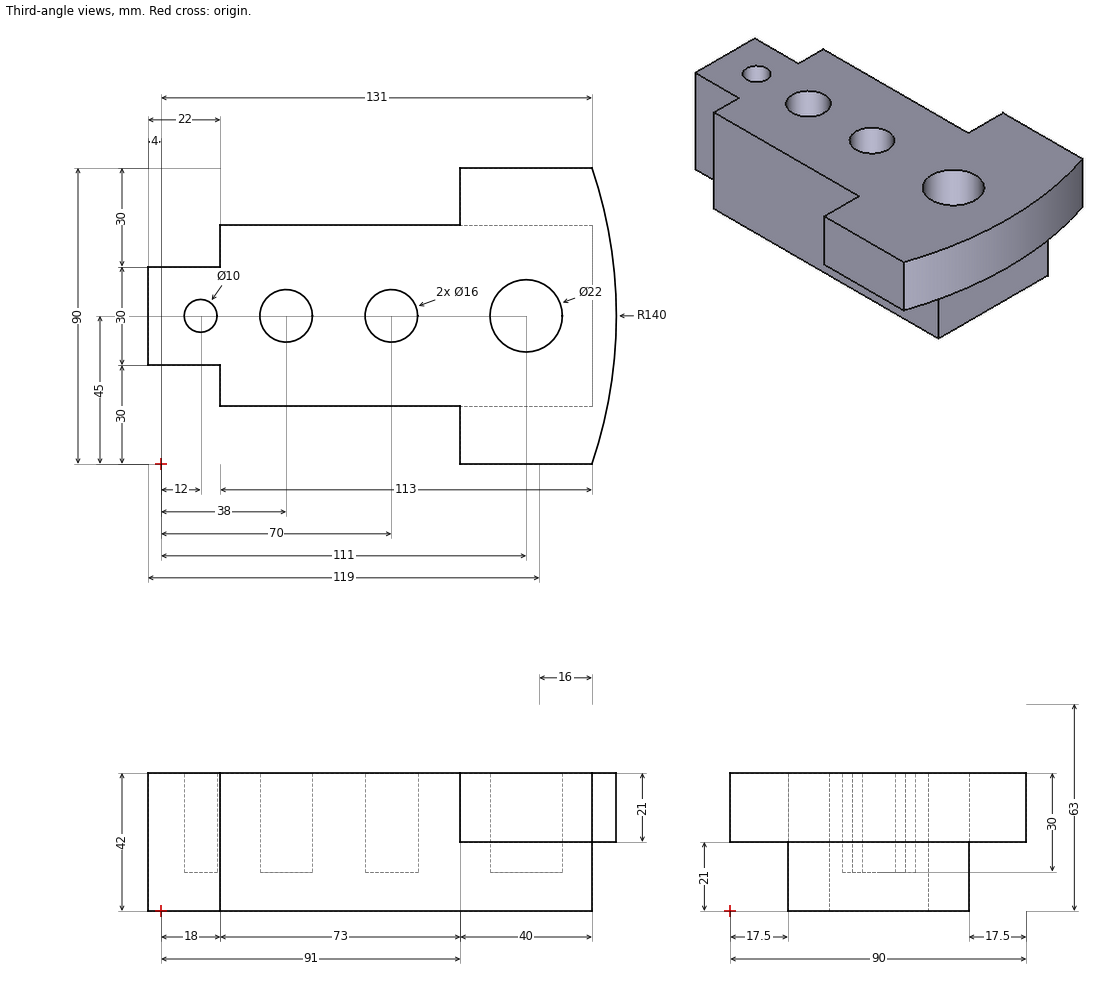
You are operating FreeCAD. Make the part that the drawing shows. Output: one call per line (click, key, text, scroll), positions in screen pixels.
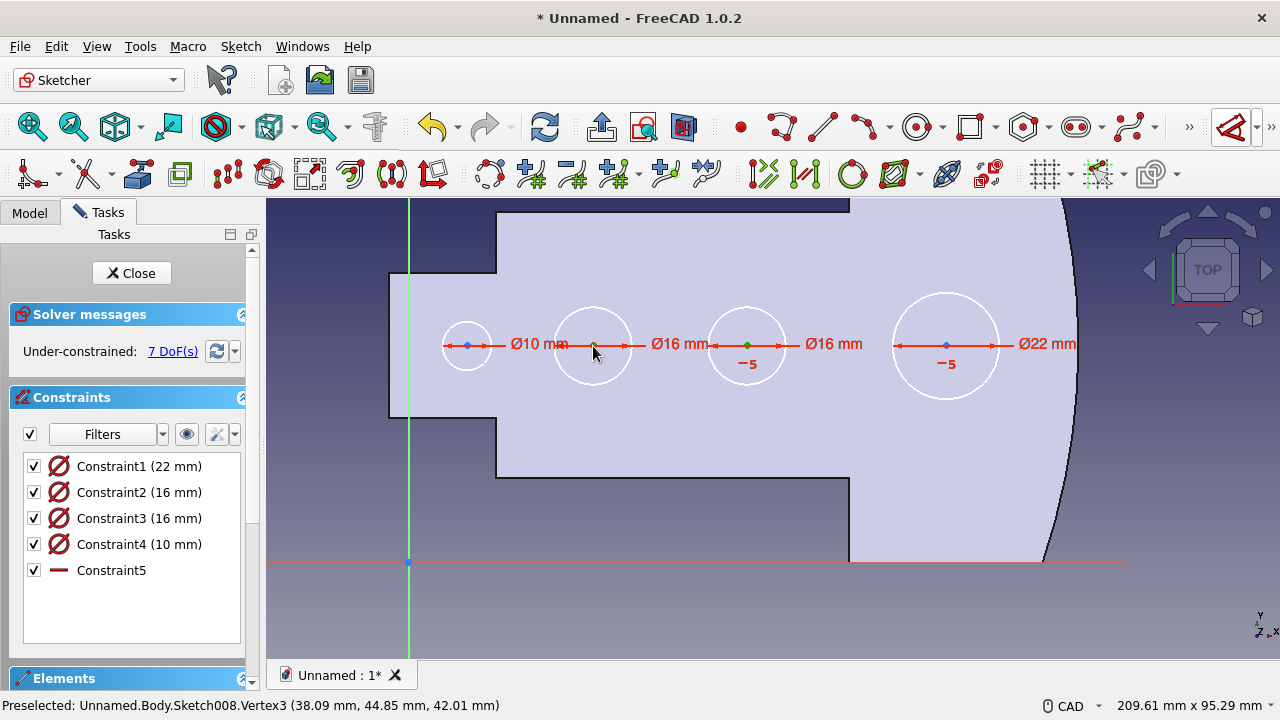
key(h)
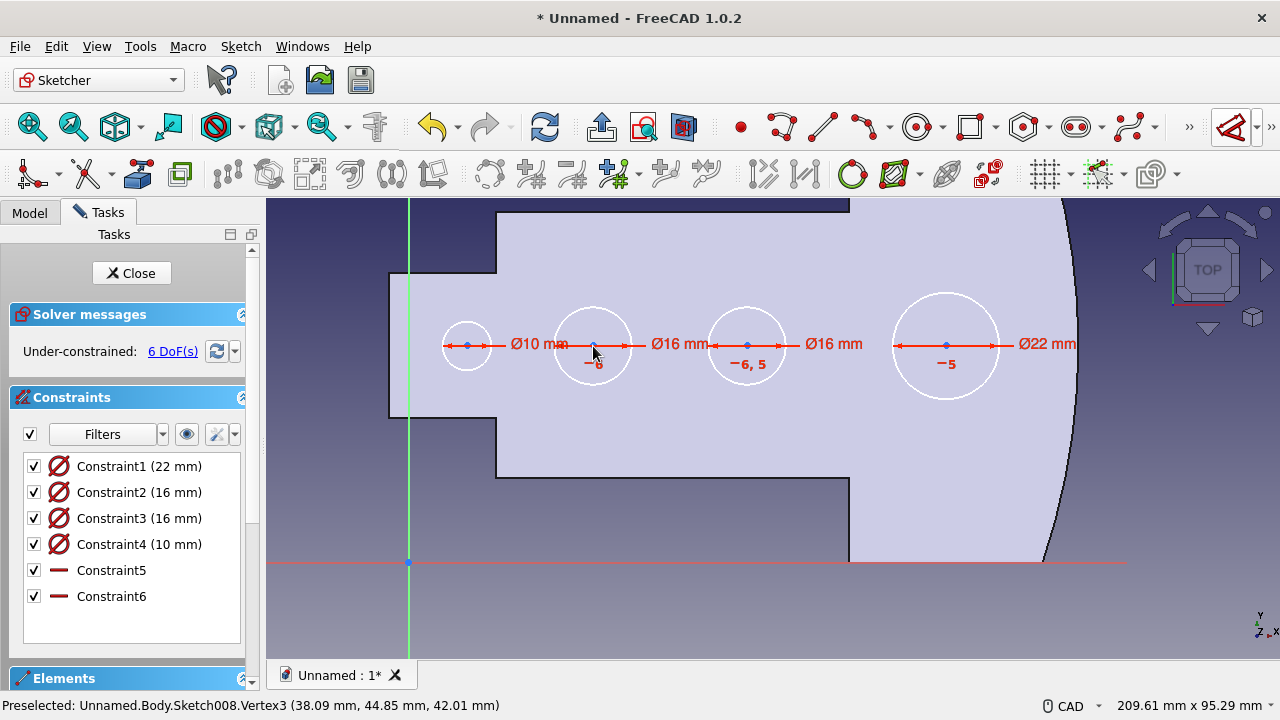
click(593, 346)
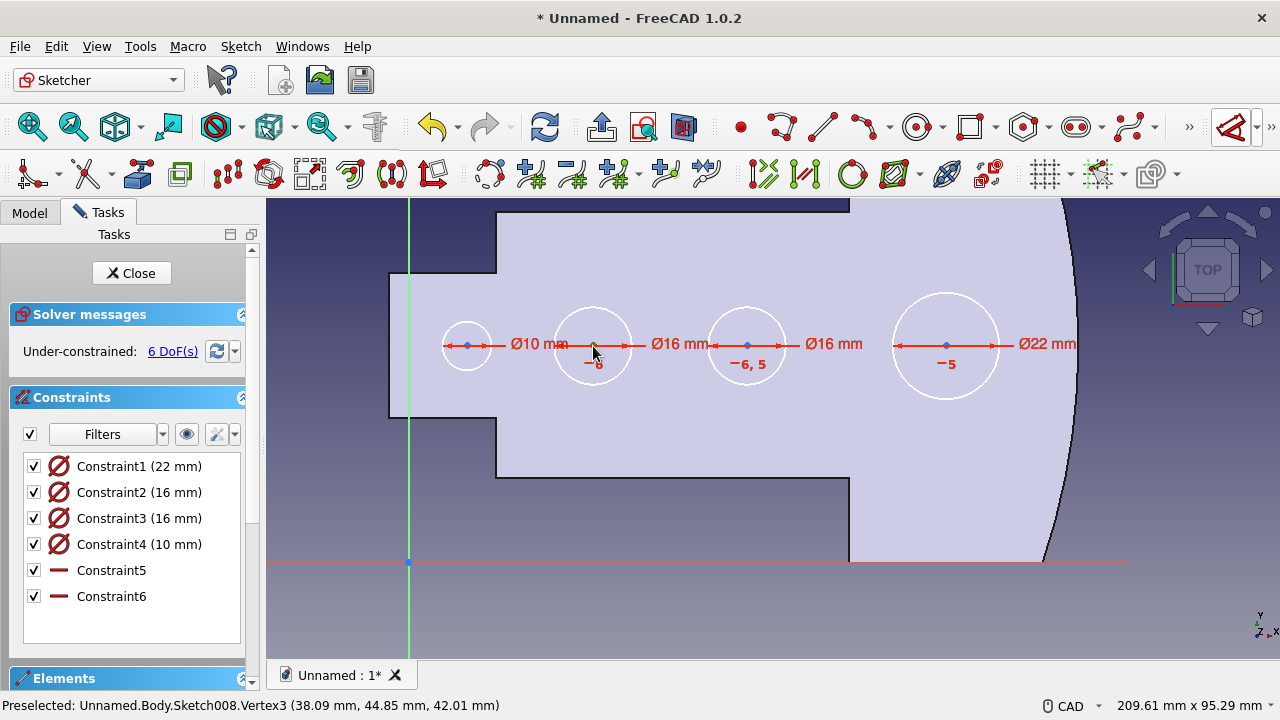
click(467, 346)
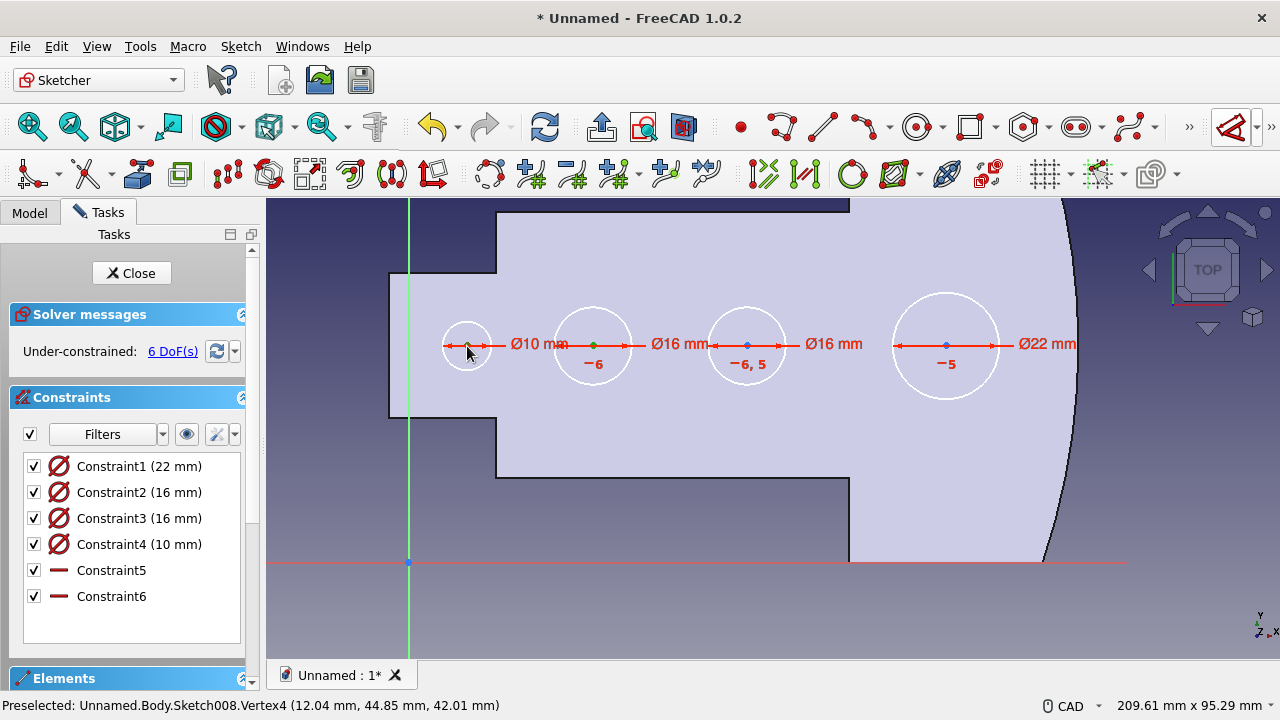
key(h)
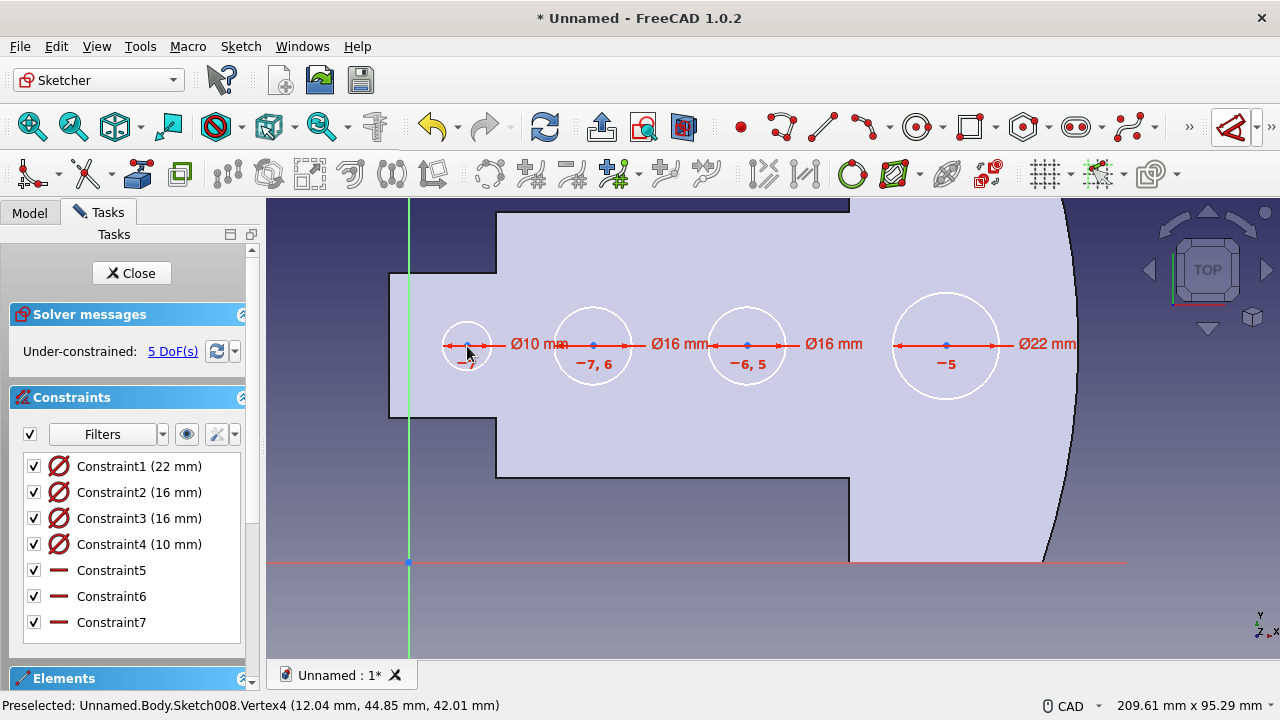
click(946, 346)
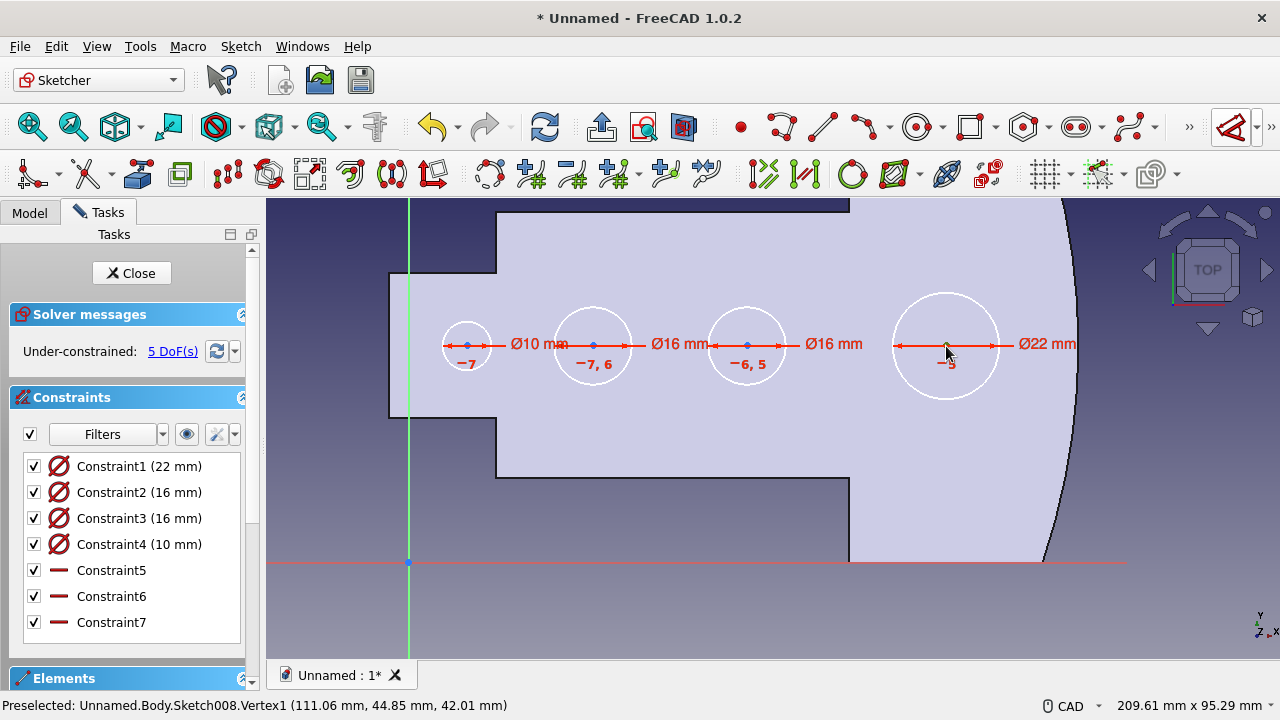
key(i)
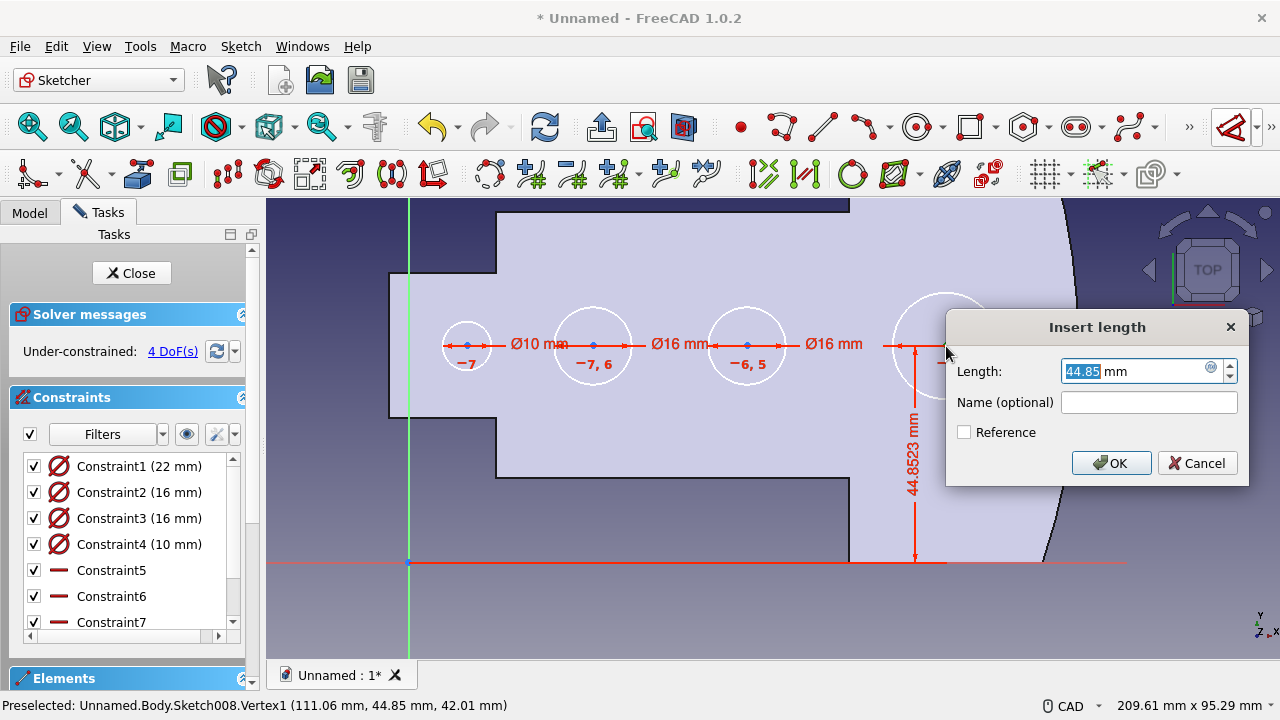
text(45)
key(Return)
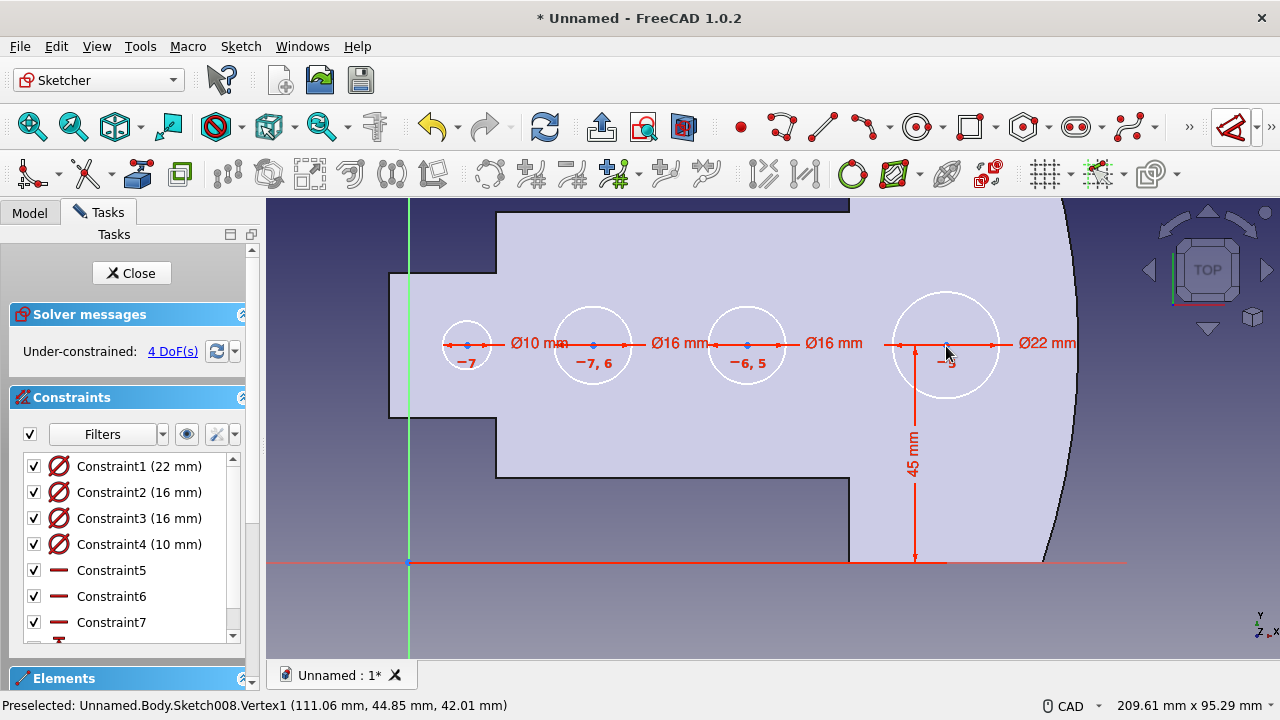
click(747, 345)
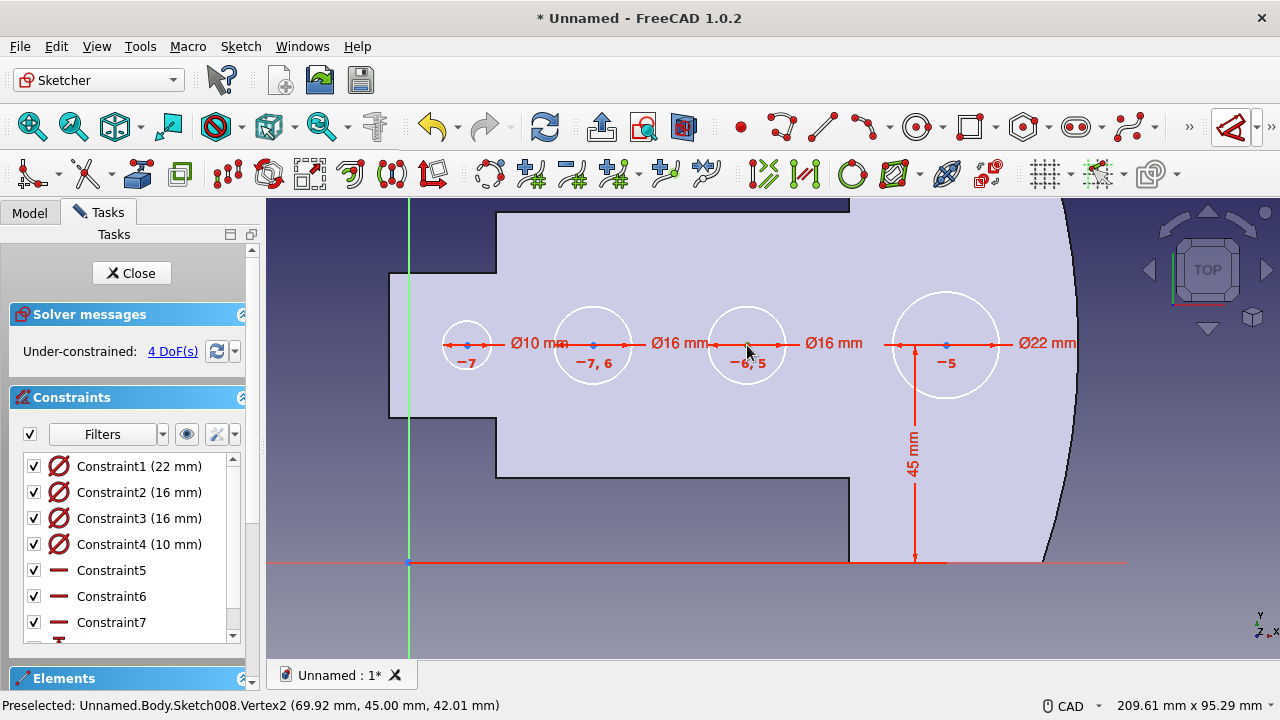
click(1256, 128)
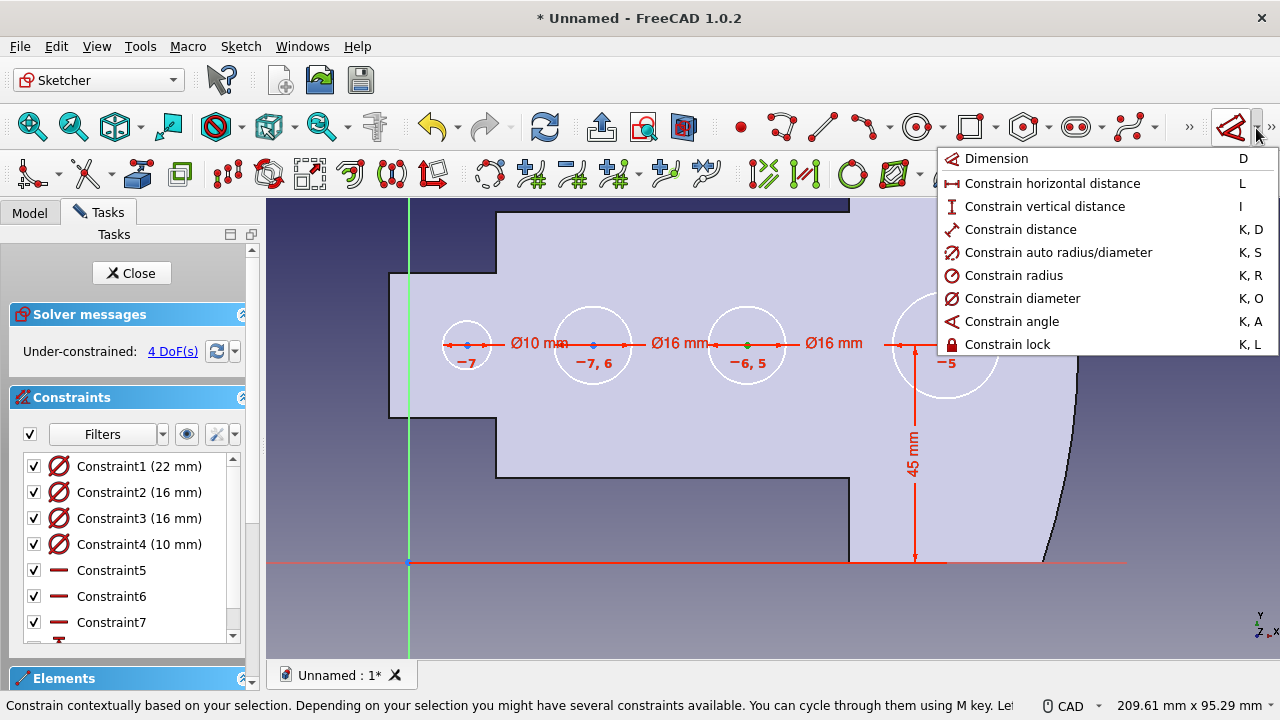
click(1108, 184)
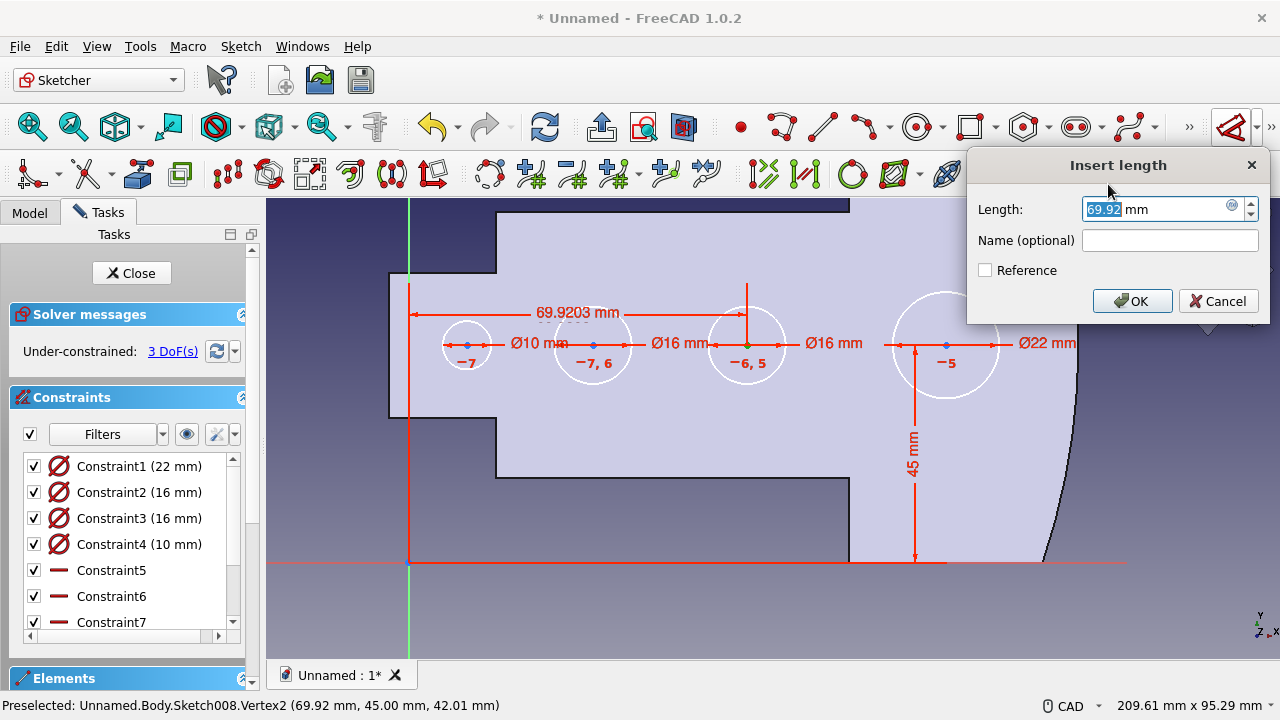
text(70)
key(Return)